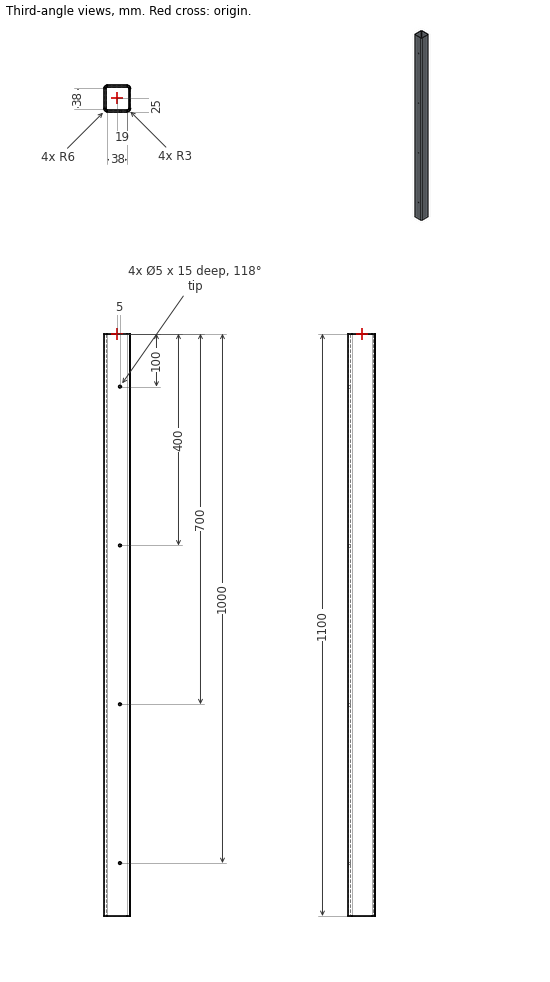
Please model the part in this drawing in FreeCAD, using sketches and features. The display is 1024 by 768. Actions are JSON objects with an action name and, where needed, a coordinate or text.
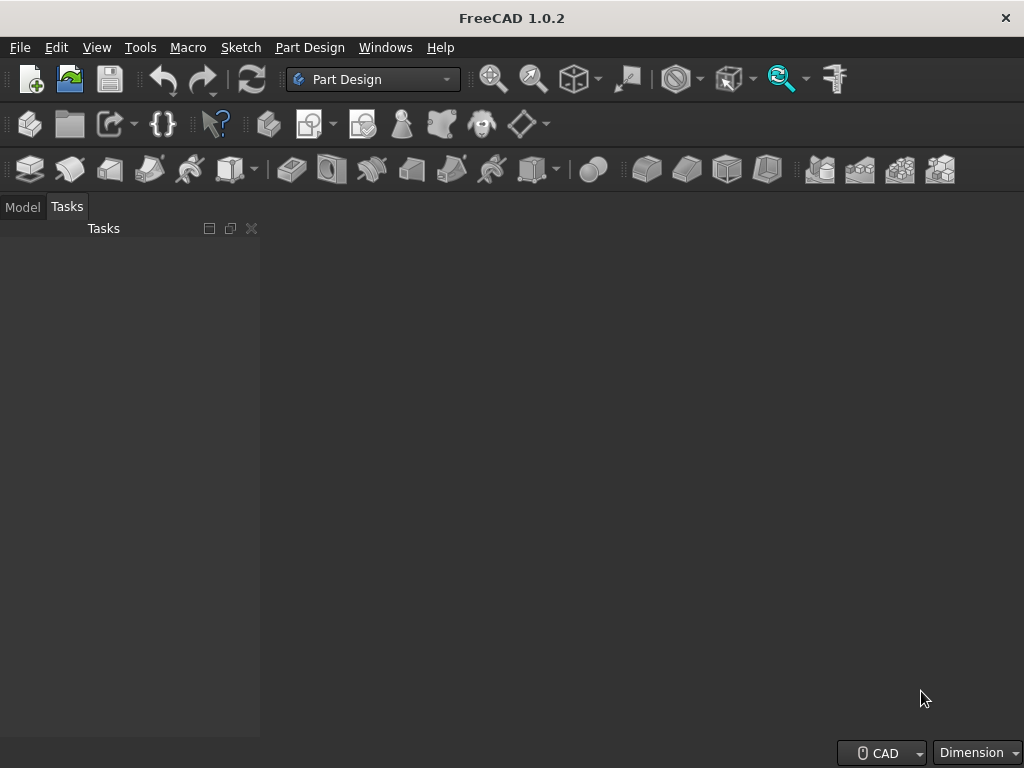
{"action": "left_click", "coordinate": [30, 80]}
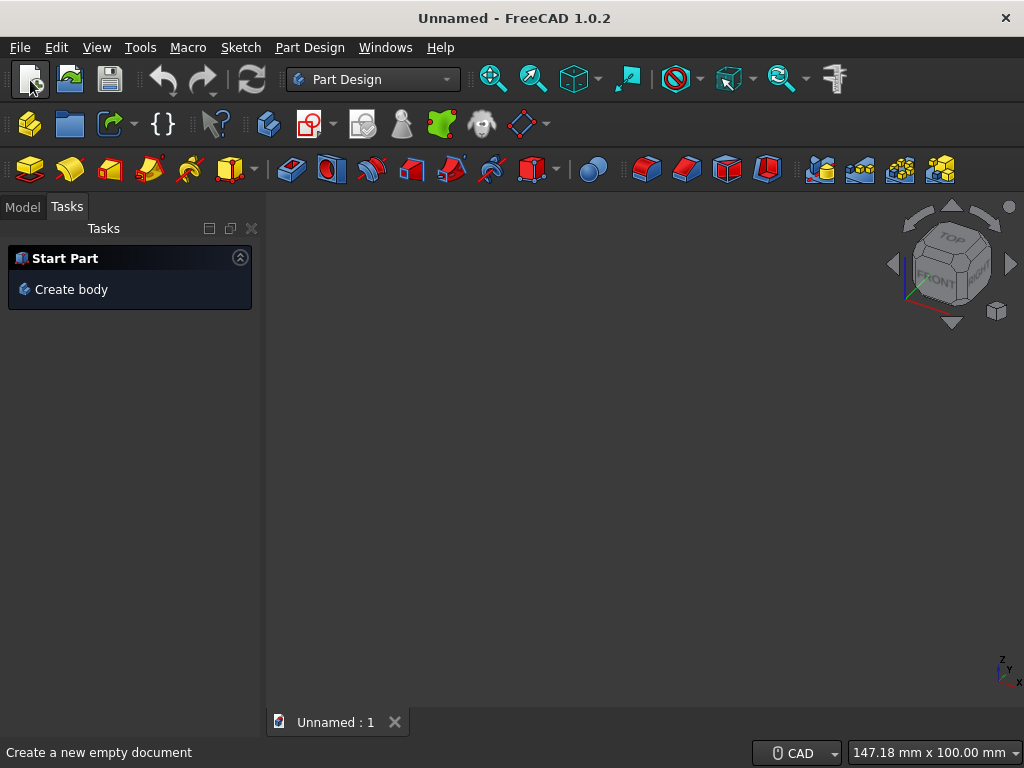
{"action": "left_click", "coordinate": [310, 124]}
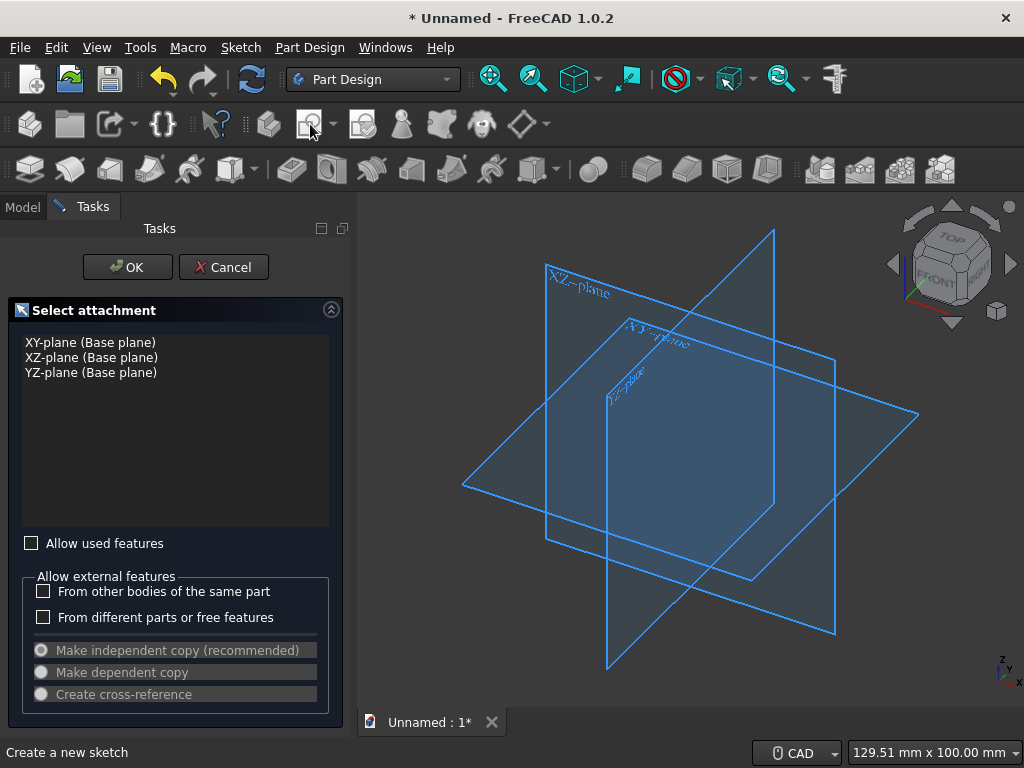
{"action": "left_click", "coordinate": [82, 342]}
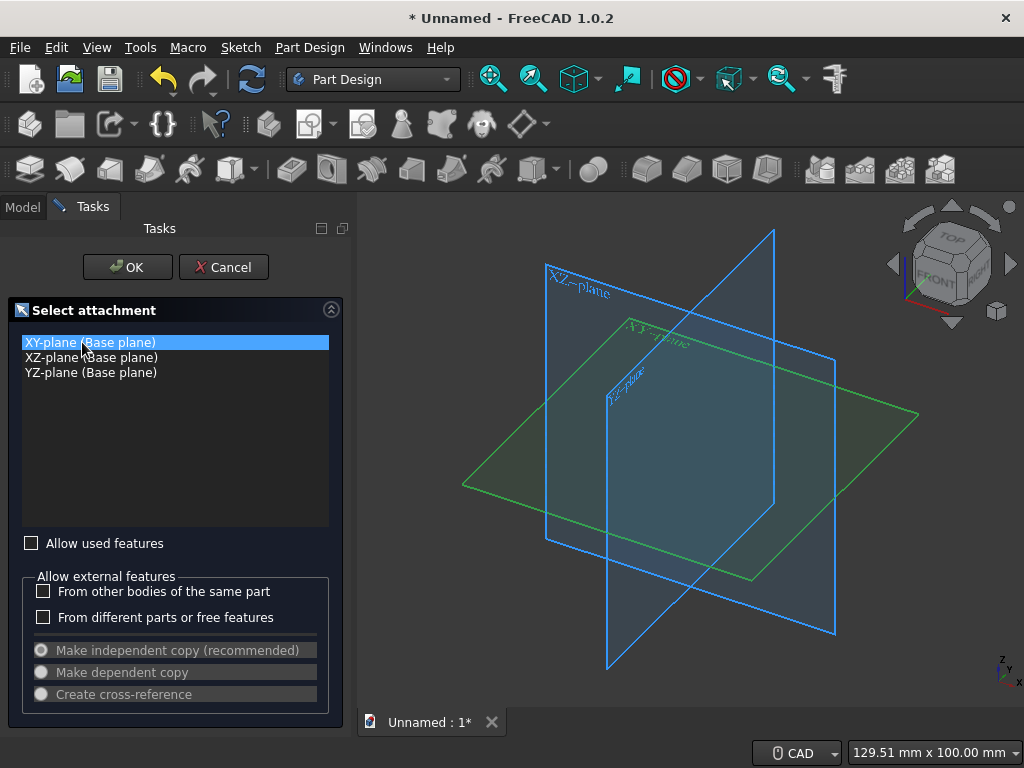
{"action": "left_click", "coordinate": [128, 267]}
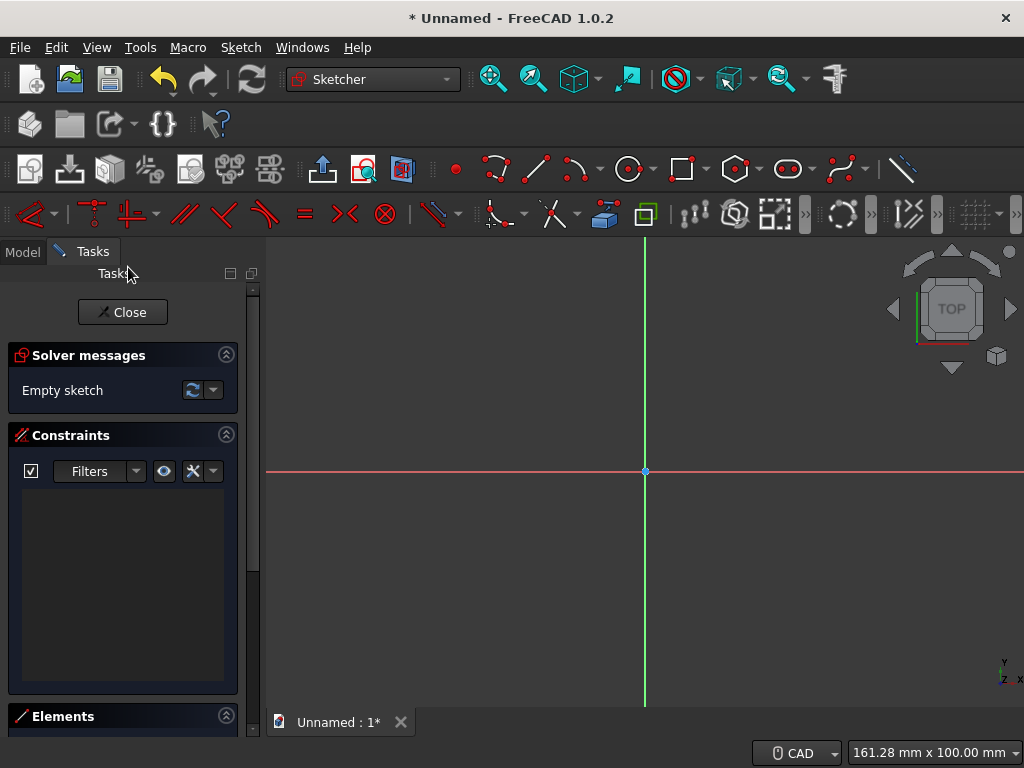
{"action": "left_click", "coordinate": [536, 170]}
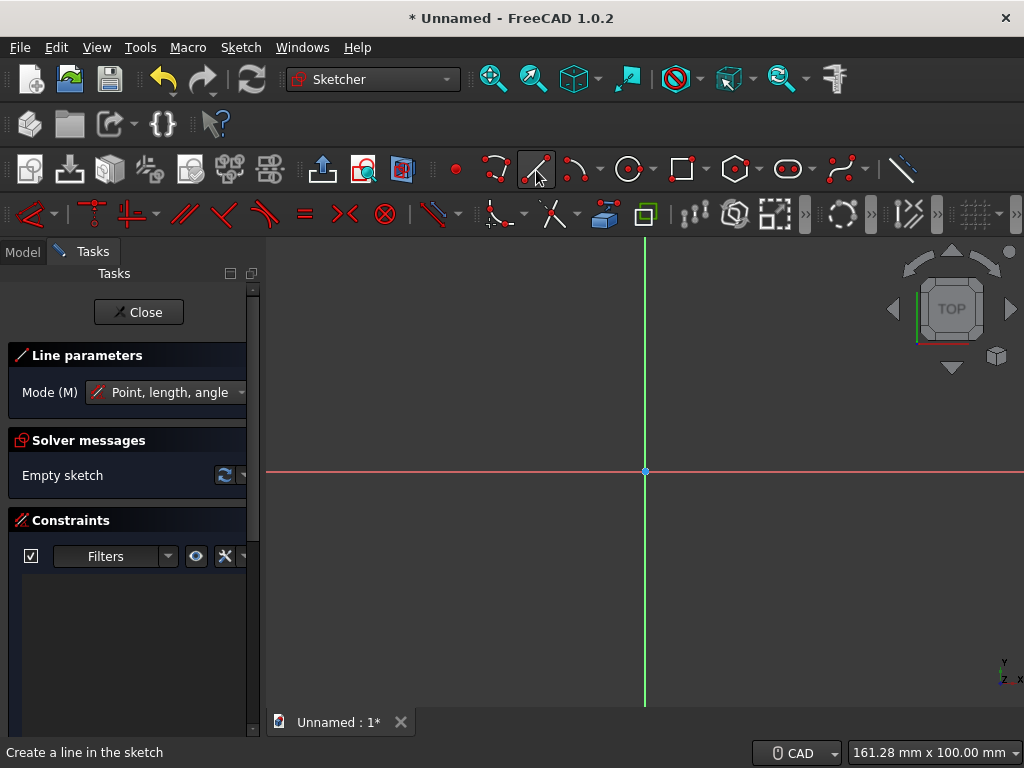
{"action": "left_click", "coordinate": [734, 590]}
{"action": "left_click", "coordinate": [556, 590]}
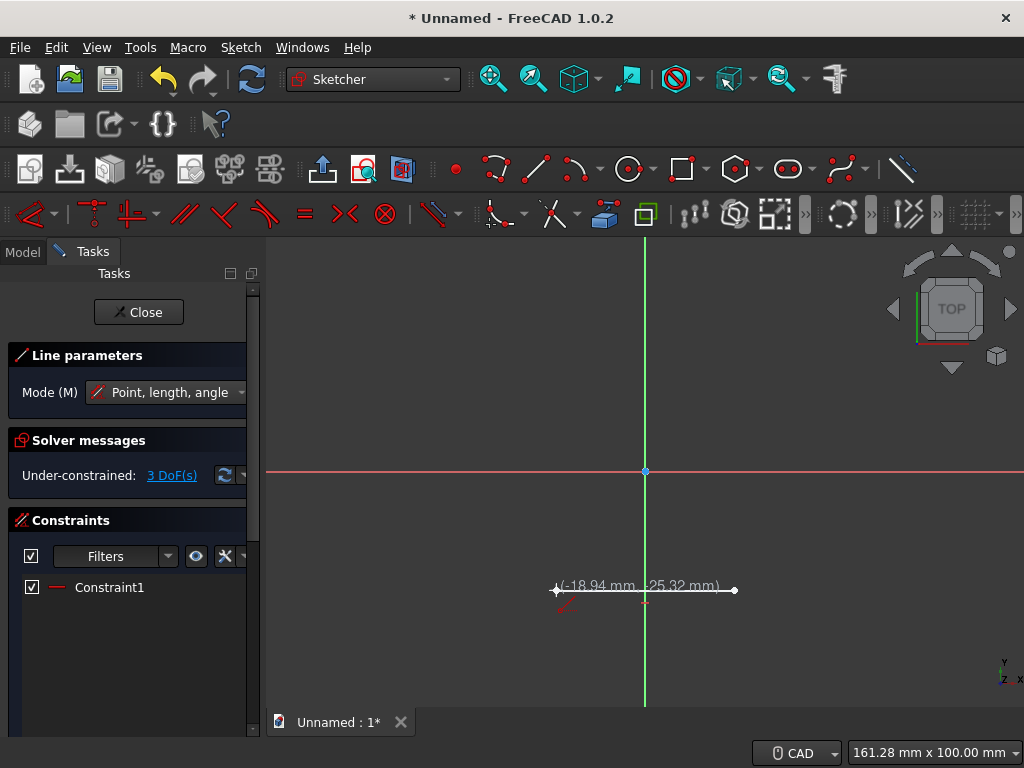
{"action": "left_click", "coordinate": [528, 561]}
{"action": "left_click", "coordinate": [528, 383]}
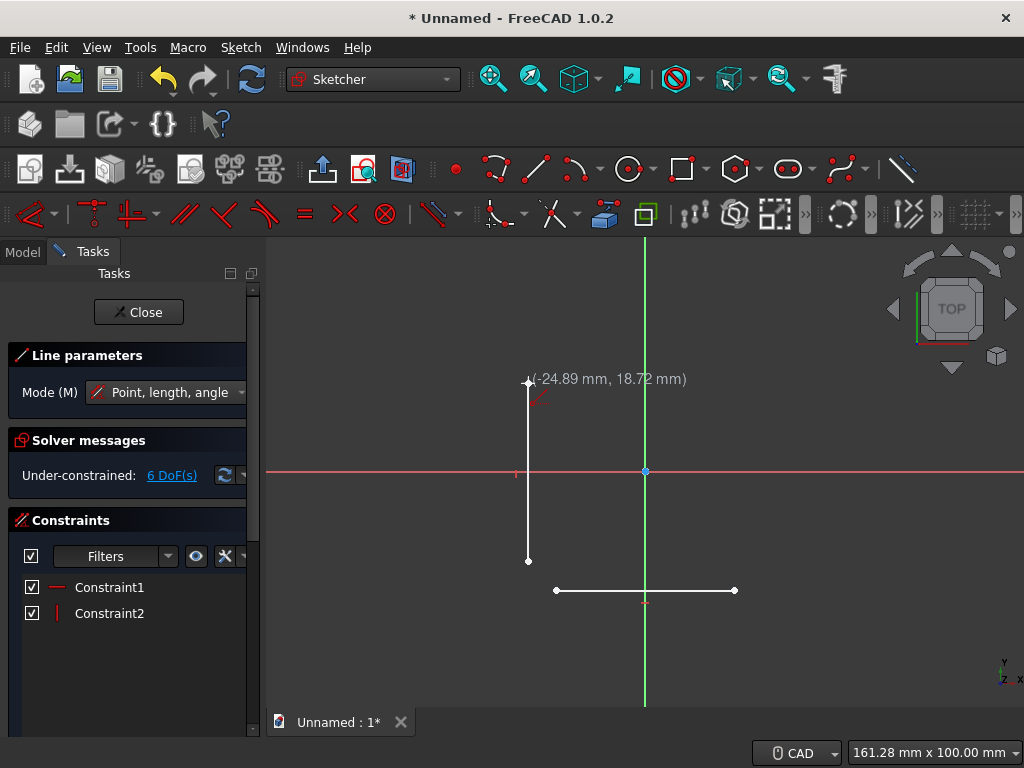
{"action": "left_click", "coordinate": [556, 354]}
{"action": "left_click", "coordinate": [734, 354]}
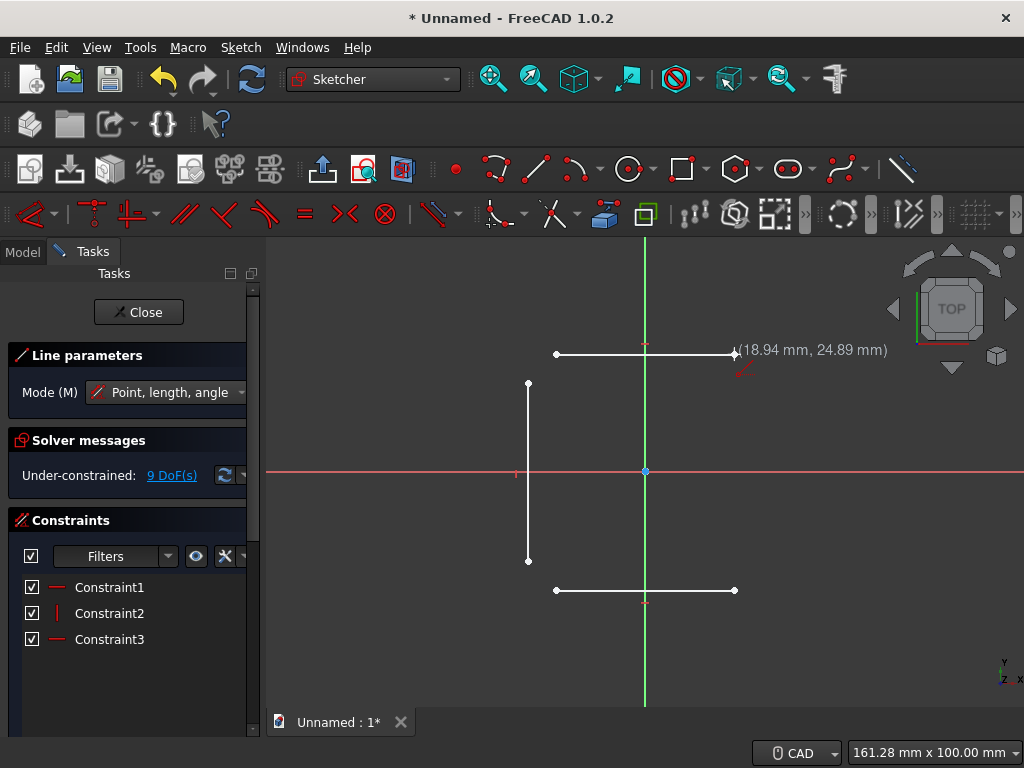
{"action": "left_click", "coordinate": [762, 383]}
{"action": "left_click", "coordinate": [762, 561]}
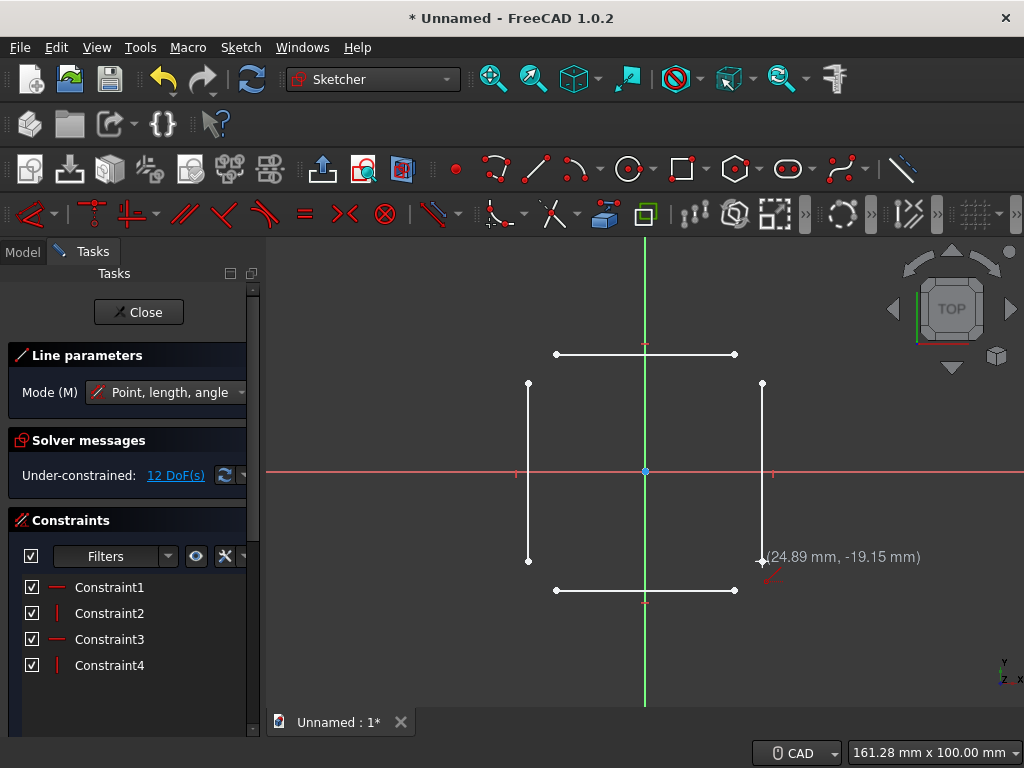
{"action": "key", "text": "g 3 a"}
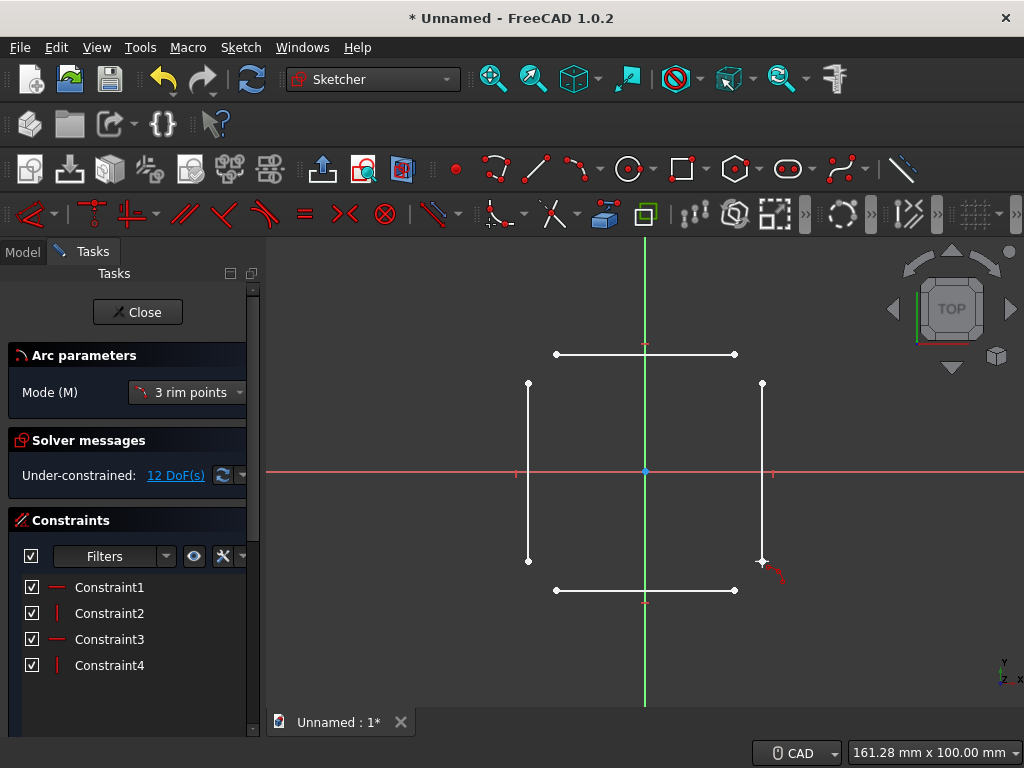
{"action": "left_click", "coordinate": [556, 591]}
{"action": "left_click", "coordinate": [528, 562]}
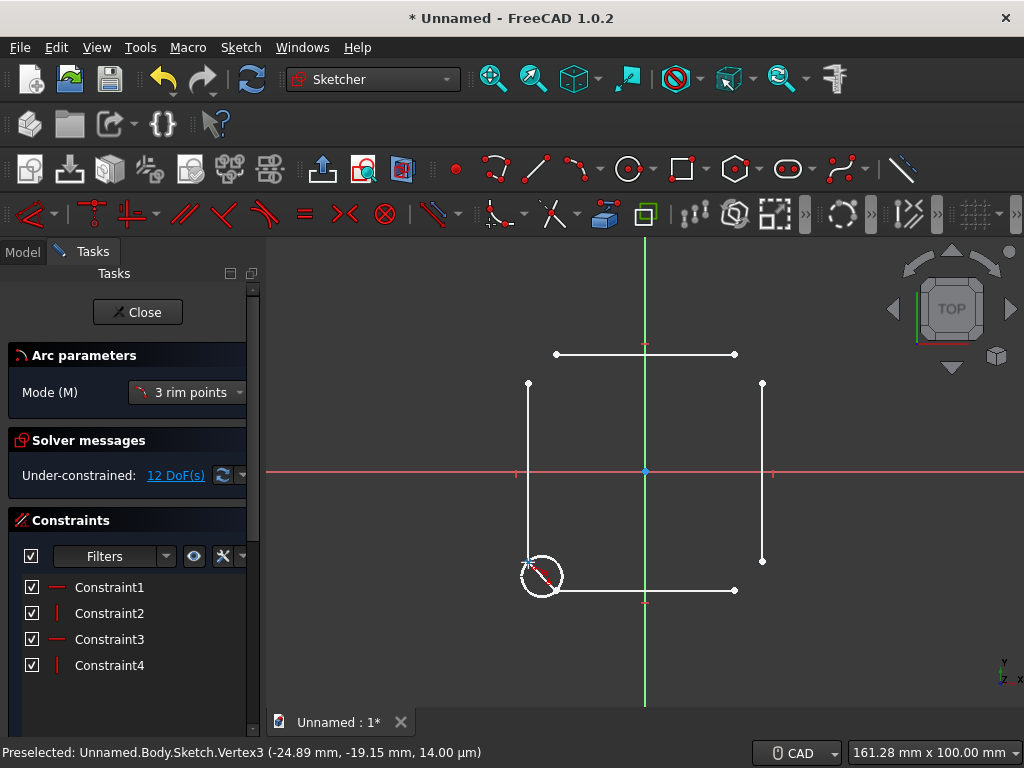
{"action": "scroll", "coordinate": [536, 581], "scroll_direction": "up", "scroll_amount": 4}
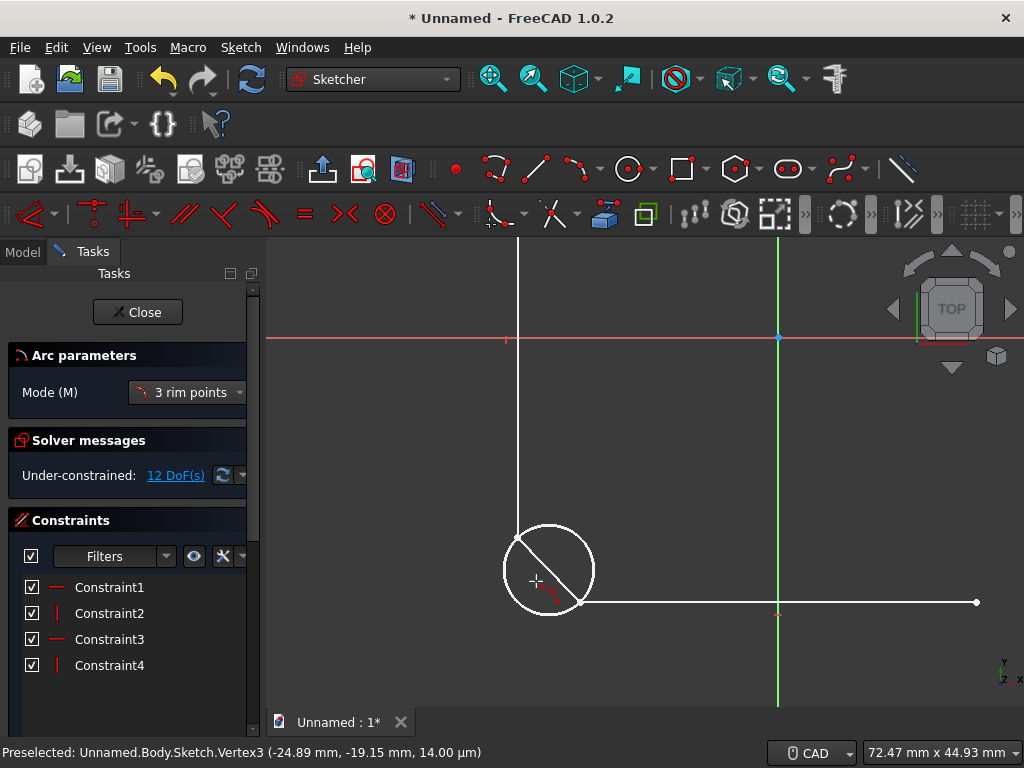
{"action": "left_click", "coordinate": [535, 581]}